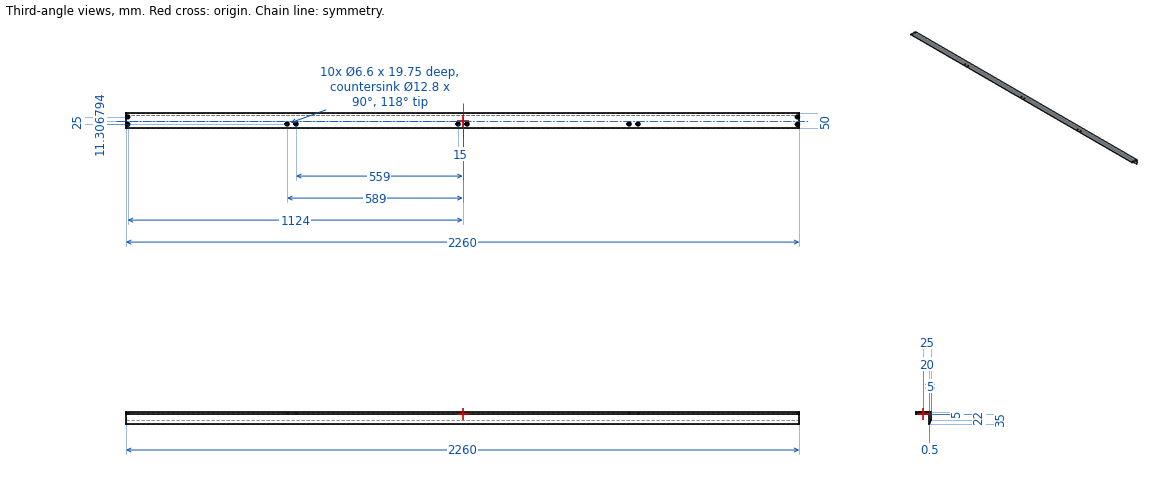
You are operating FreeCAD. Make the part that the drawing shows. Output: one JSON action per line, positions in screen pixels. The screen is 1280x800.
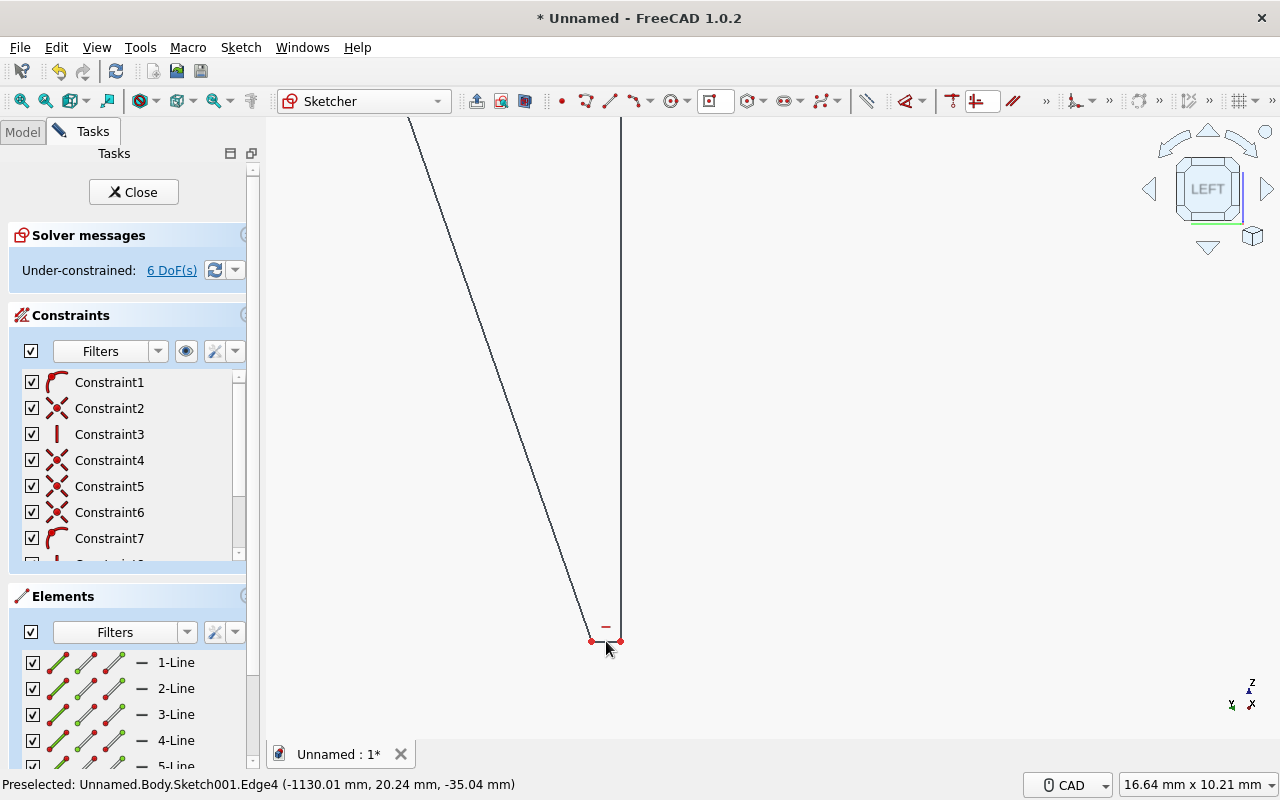
{"action": "left_click", "coordinate": [906, 102]}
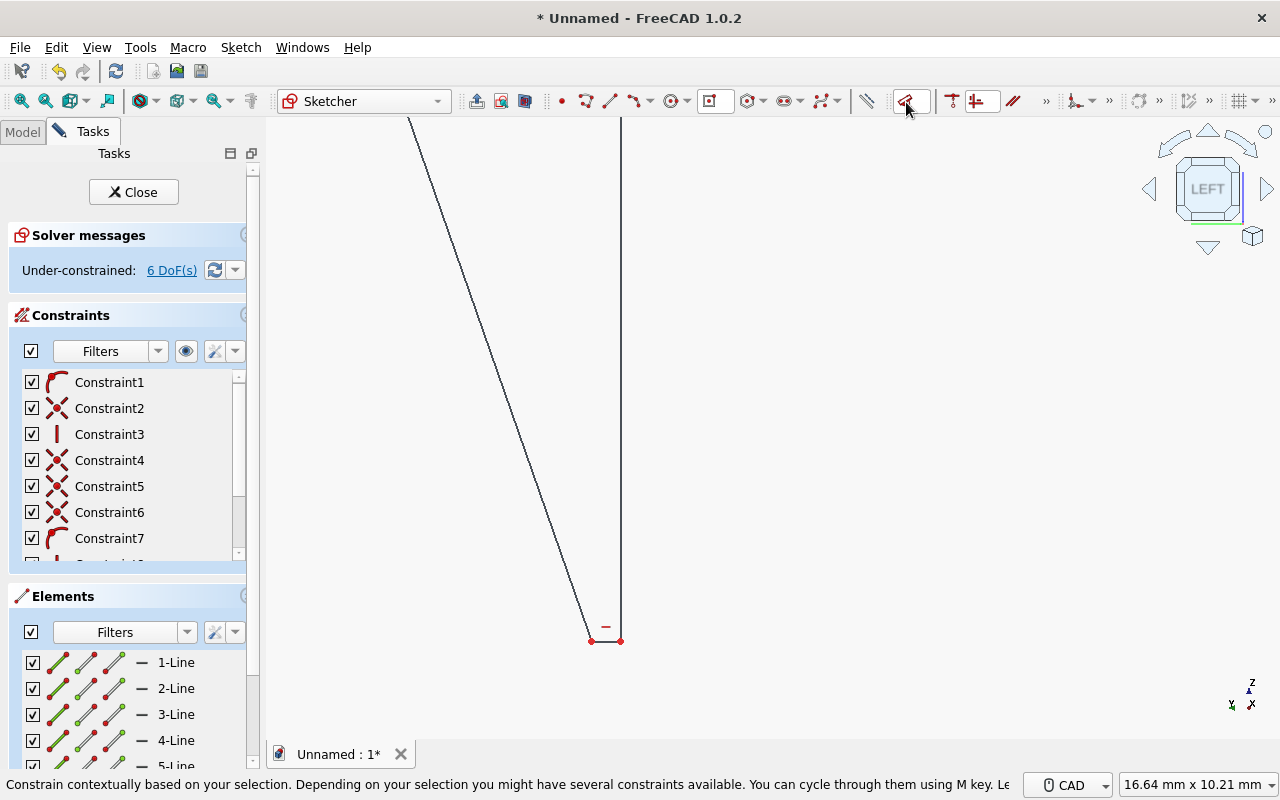
{"action": "scroll", "coordinate": [610, 644], "scroll_direction": "down", "scroll_amount": 8}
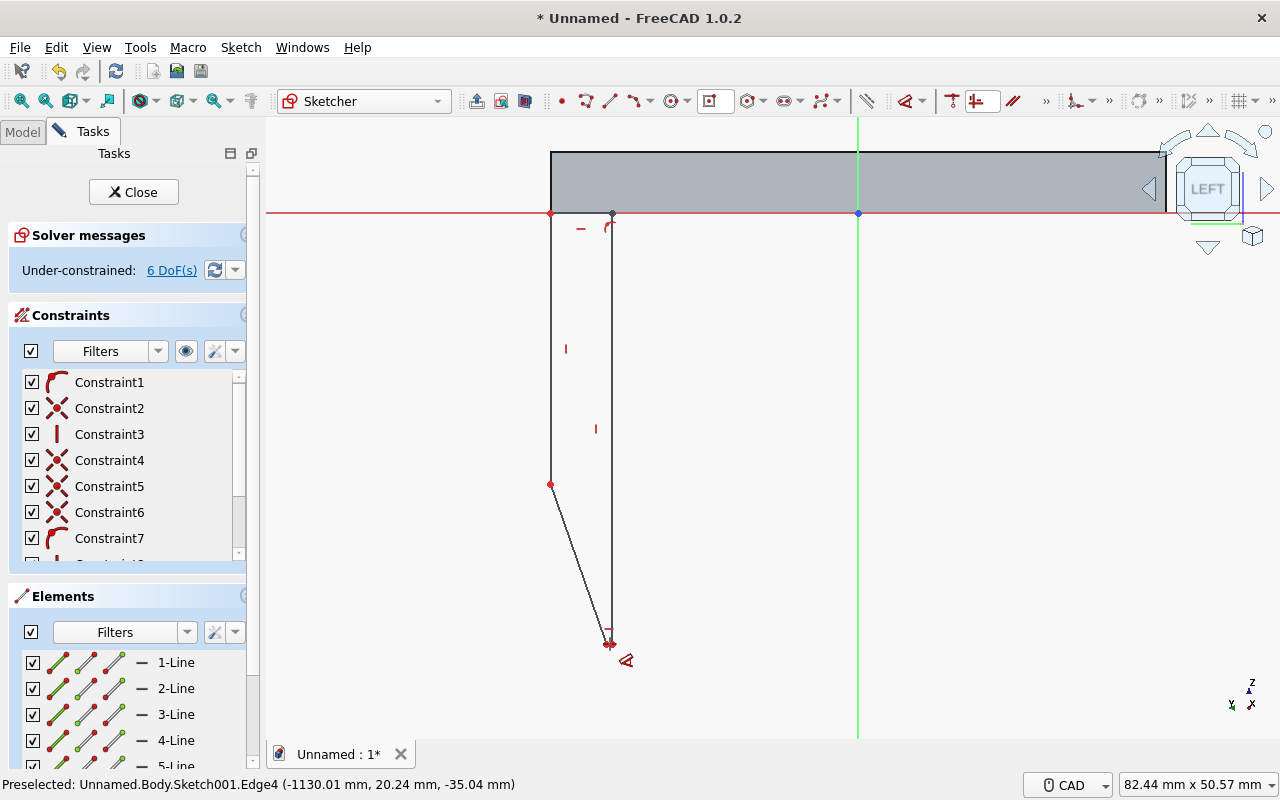
{"action": "left_click", "coordinate": [594, 213]}
{"action": "left_click", "coordinate": [582, 179]}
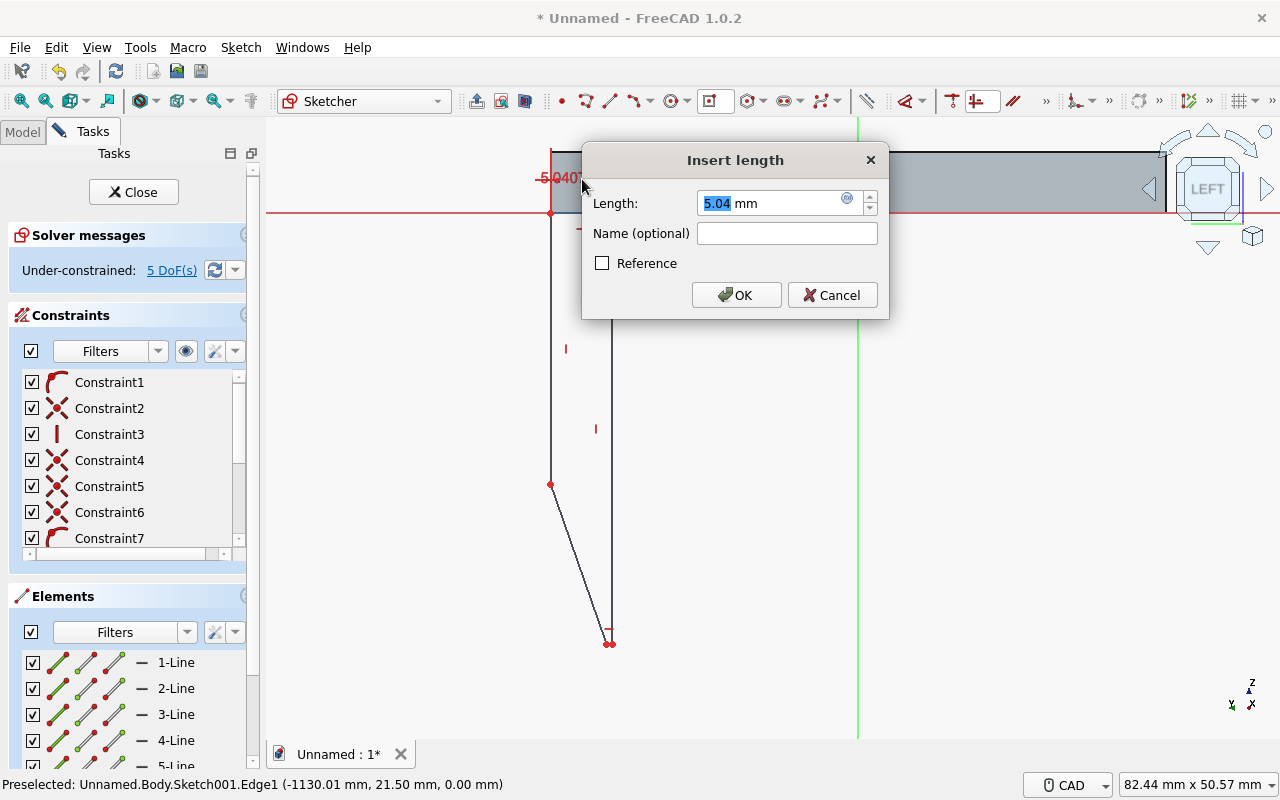
{"action": "type", "text": "5"}
{"action": "key", "text": "Return"}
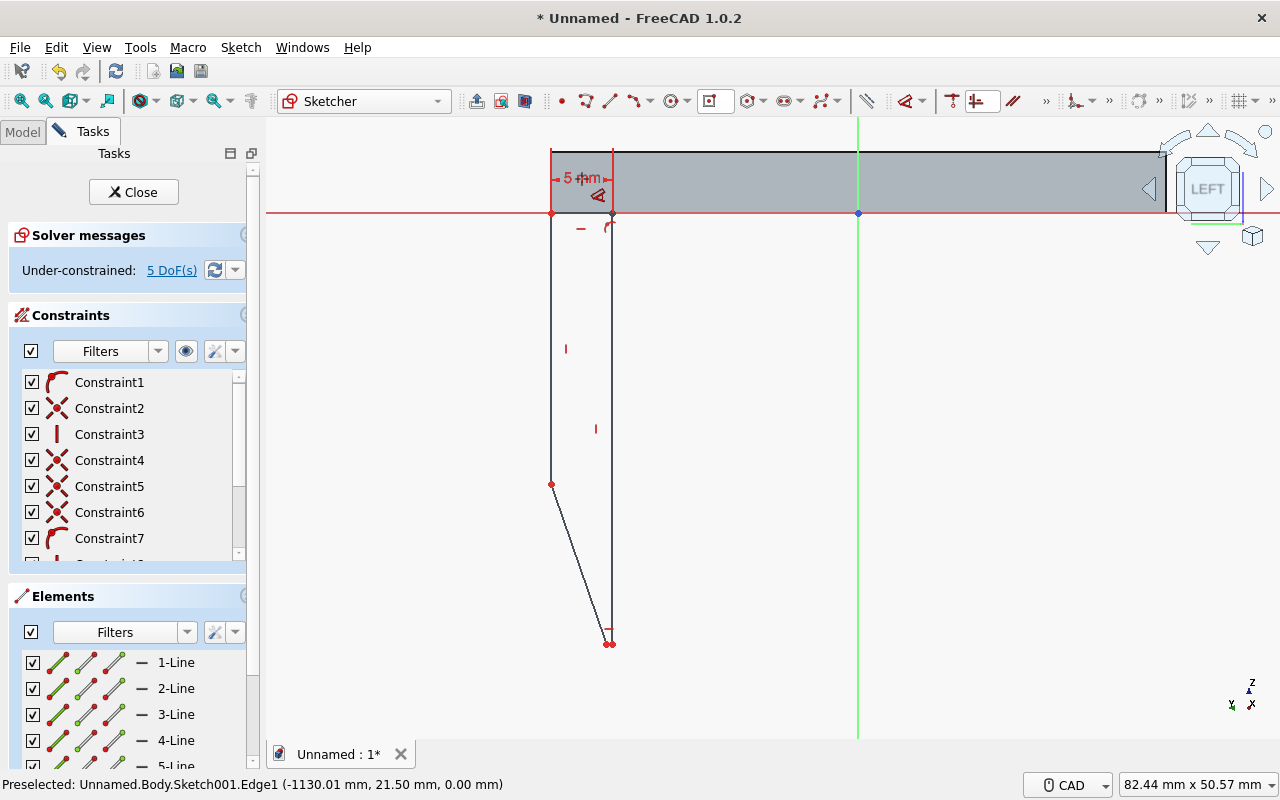
{"action": "left_click", "coordinate": [551, 294]}
{"action": "left_click", "coordinate": [517, 349]}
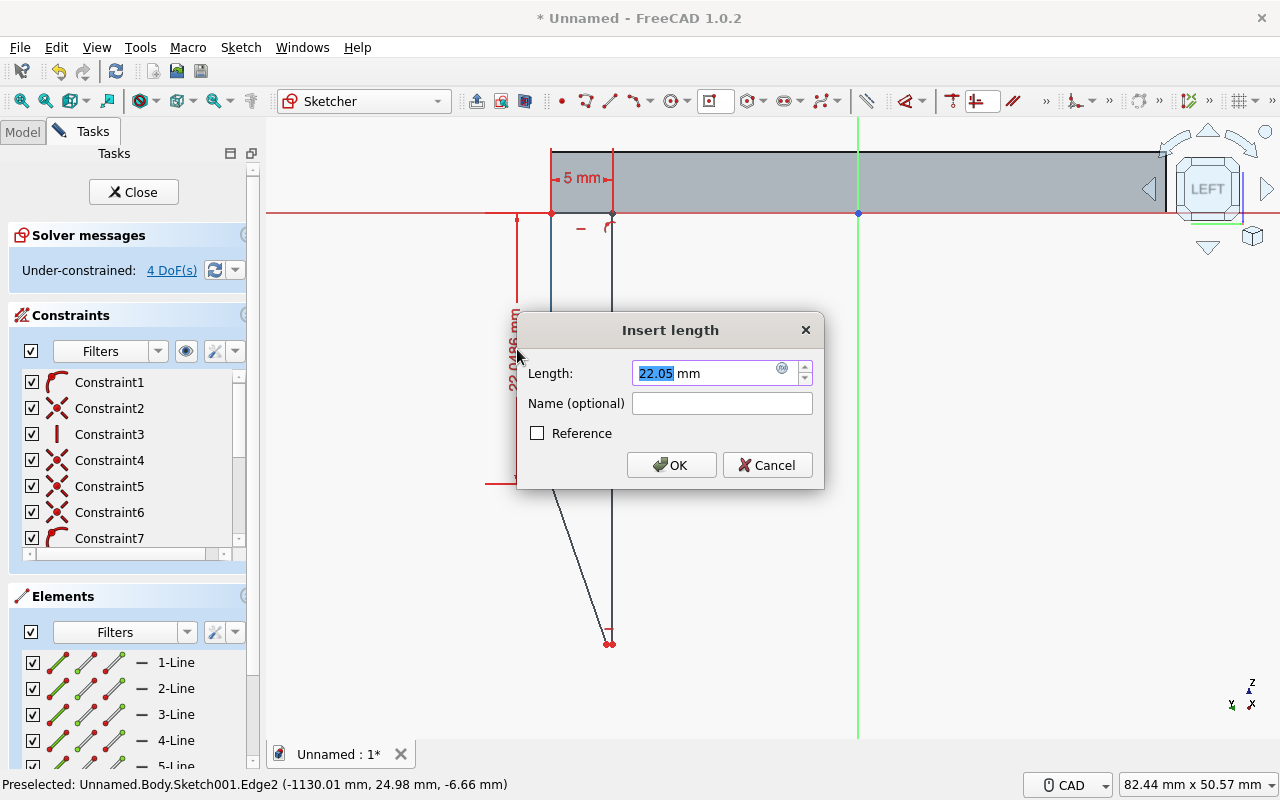
{"action": "type", "text": "22"}
{"action": "key", "text": "Return"}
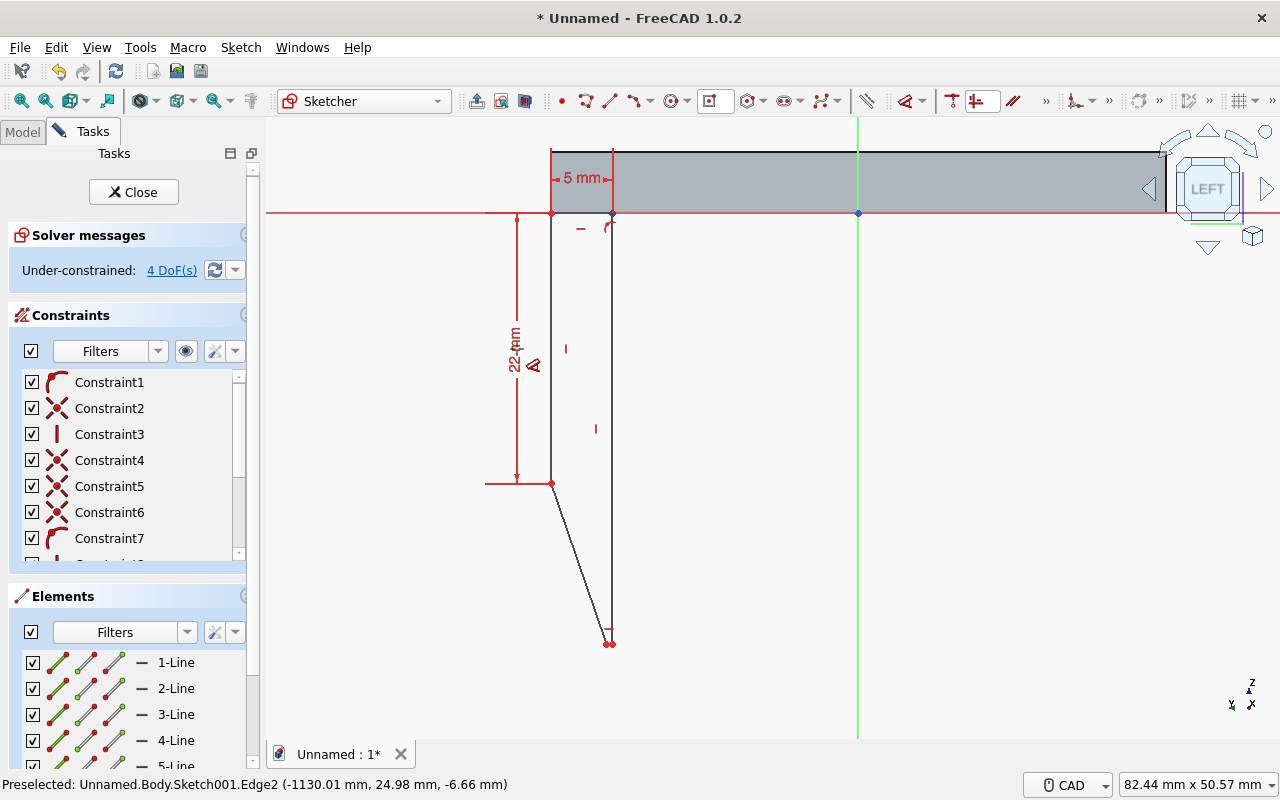
{"action": "left_click", "coordinate": [612, 515]}
{"action": "left_click", "coordinate": [578, 429]}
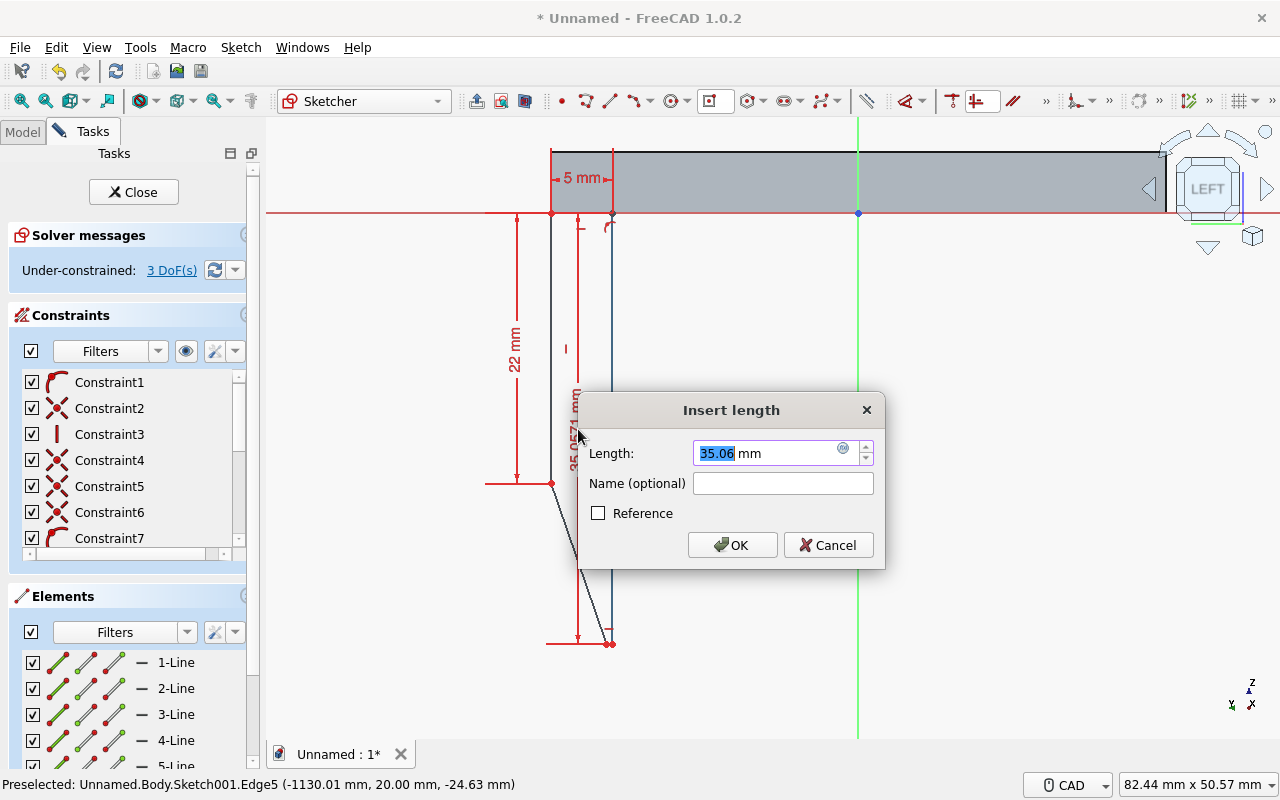
{"action": "type", "text": "35"}
{"action": "key", "text": "Return"}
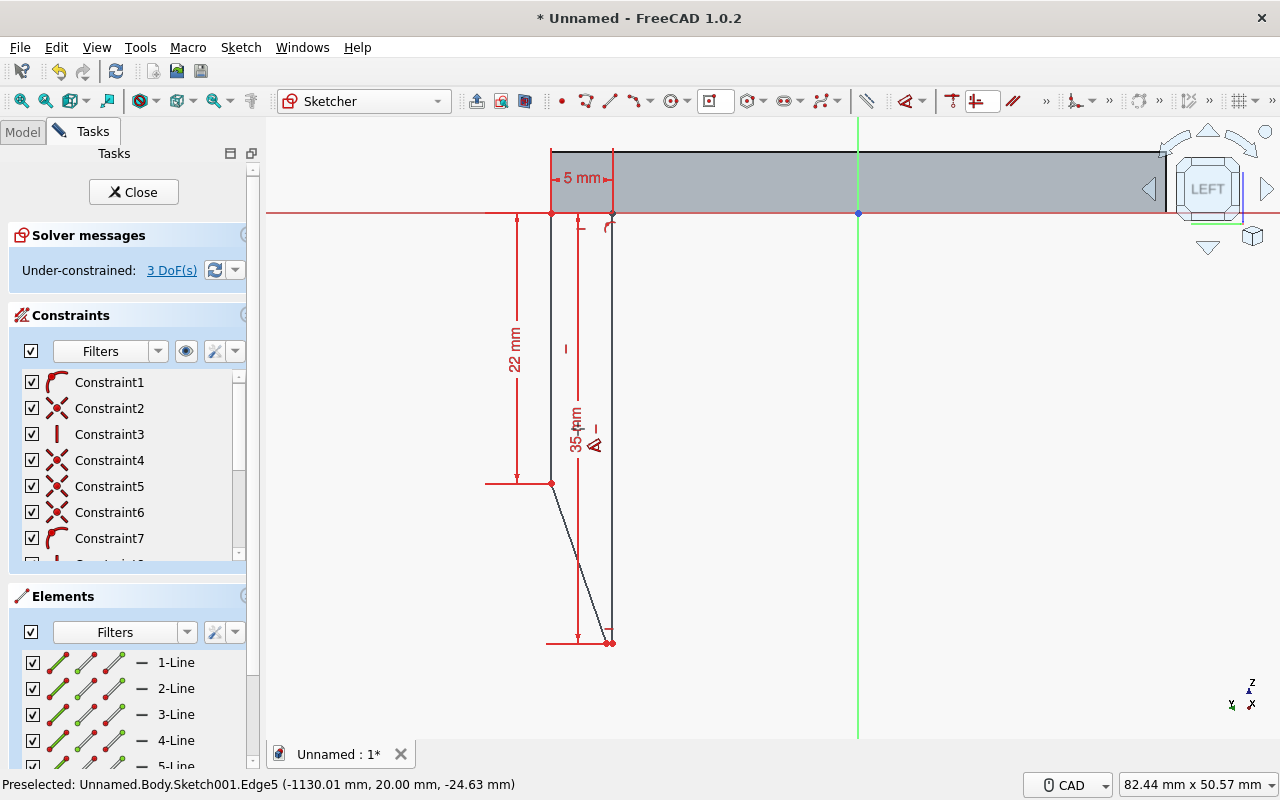
{"action": "scroll", "coordinate": [610, 644], "scroll_direction": "up", "scroll_amount": 10}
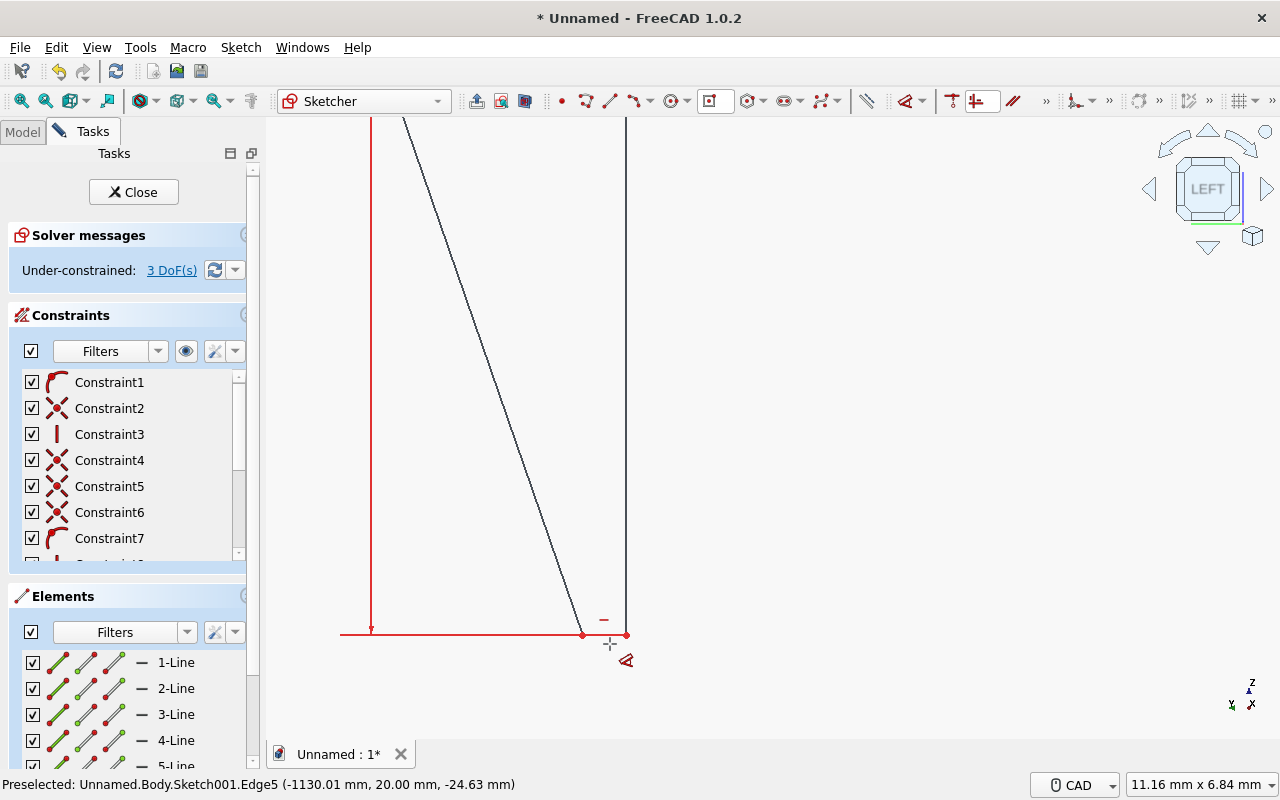
{"action": "left_click", "coordinate": [605, 635]}
{"action": "left_click", "coordinate": [605, 669]}